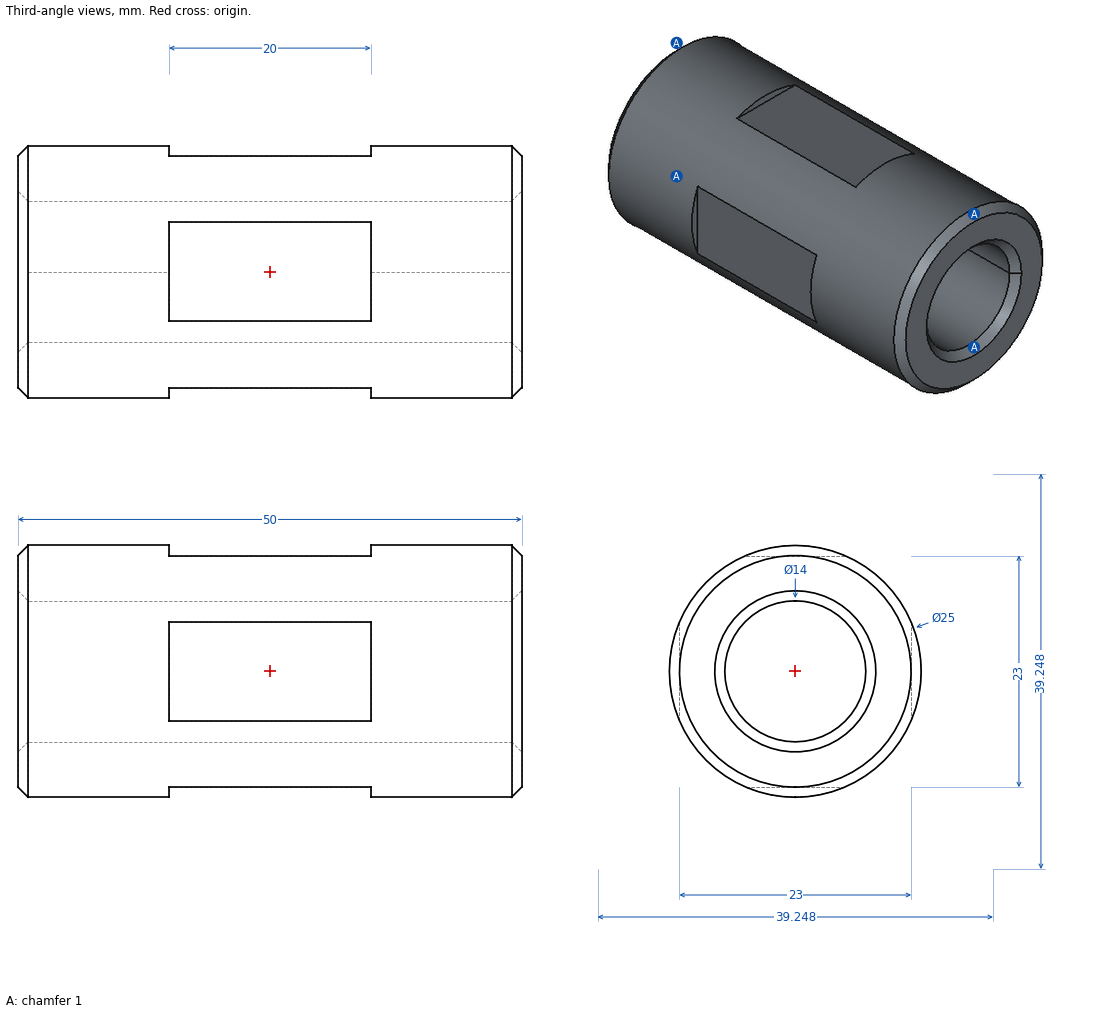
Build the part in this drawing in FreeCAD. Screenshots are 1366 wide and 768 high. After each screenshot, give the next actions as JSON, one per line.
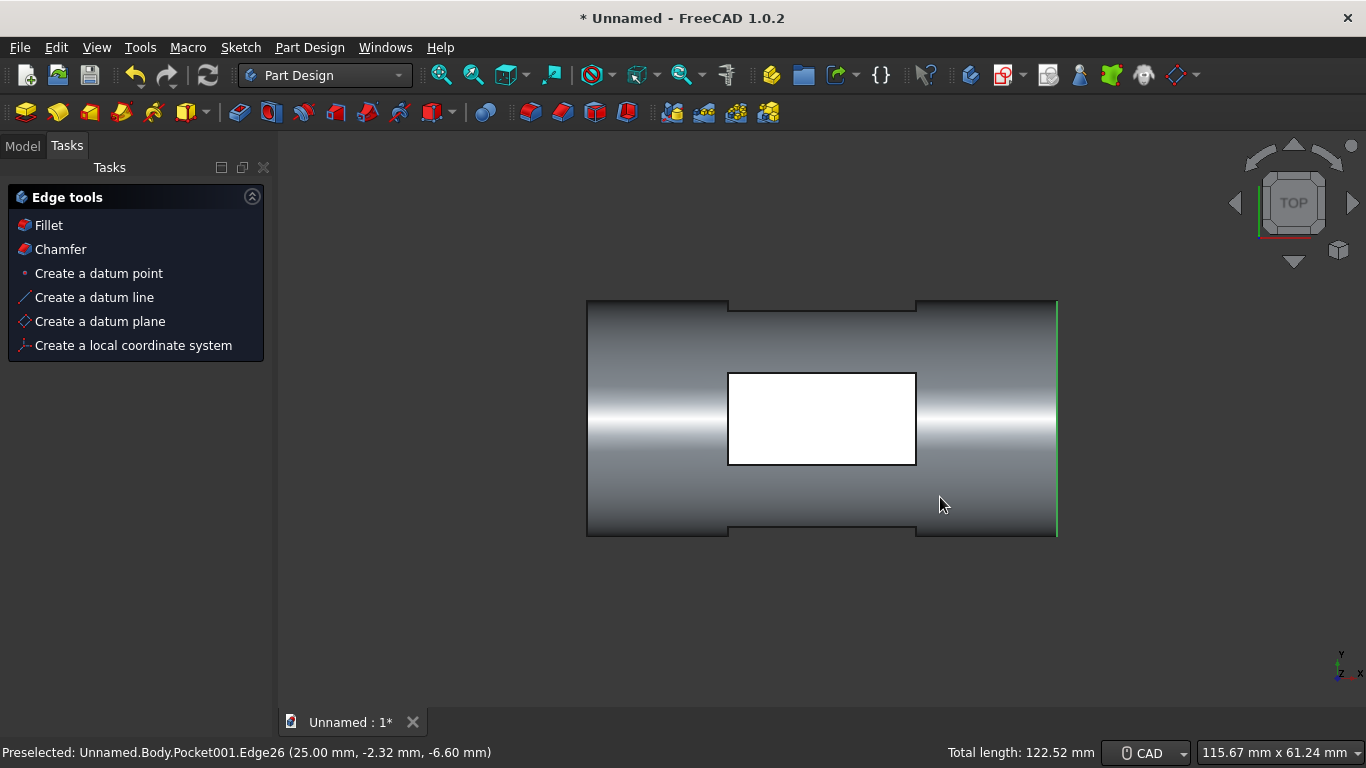
{"action": "left_click", "coordinate": [587, 513], "text": "ctrl"}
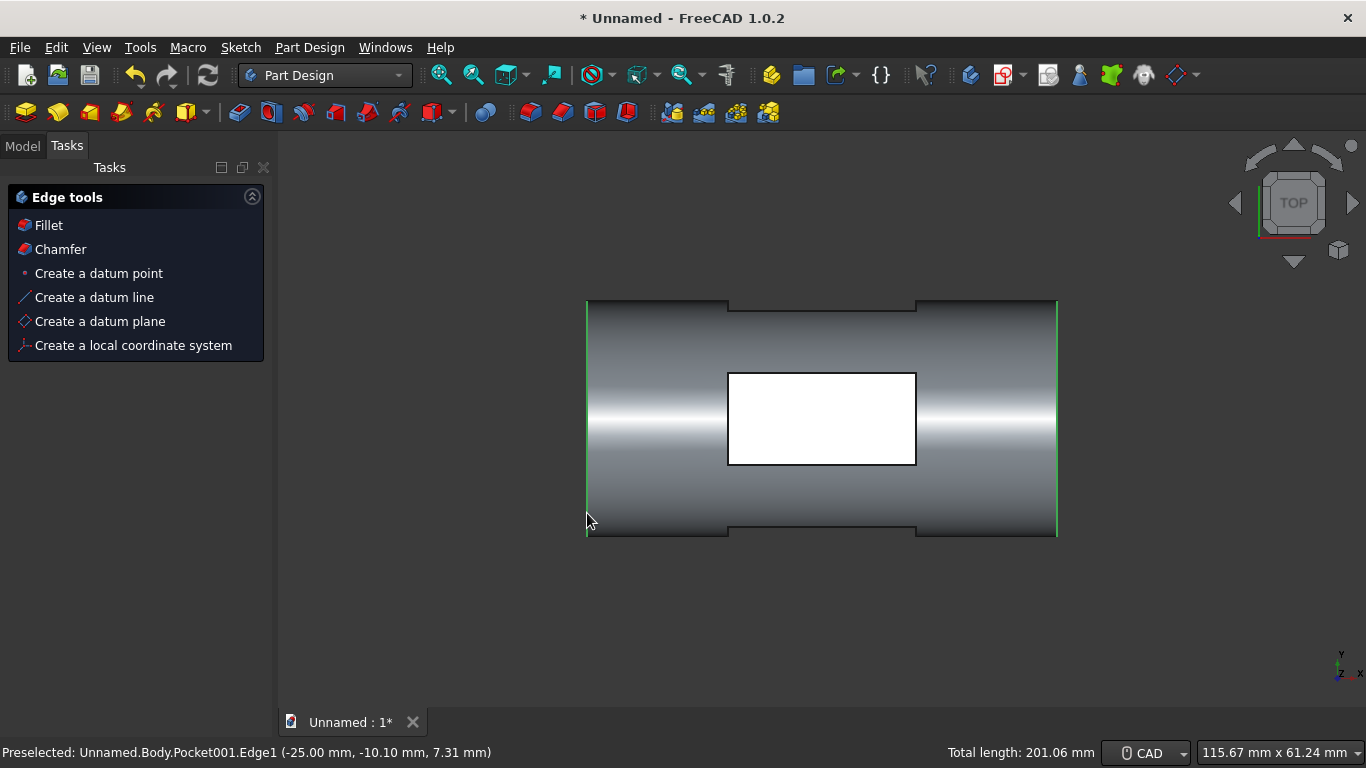
{"action": "key", "text": "1"}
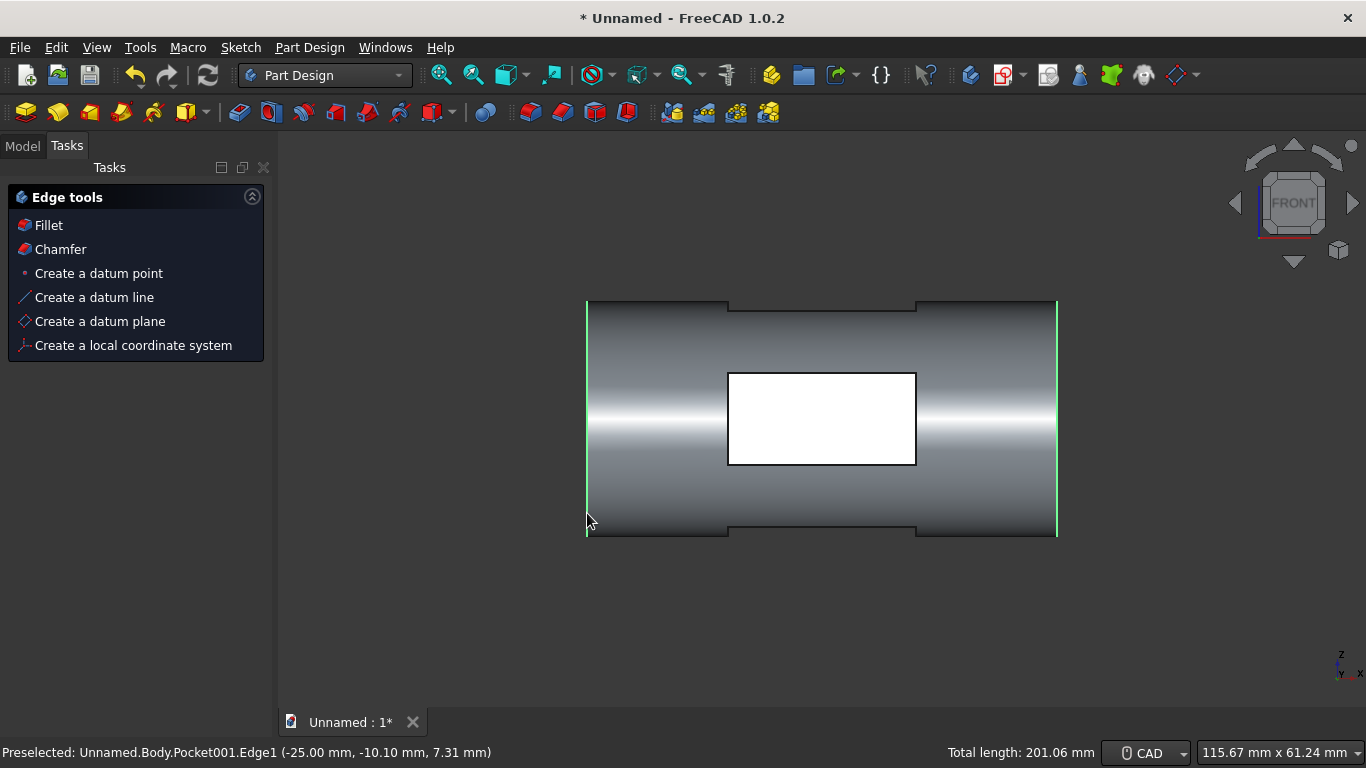
{"action": "left_click", "coordinate": [442, 76]}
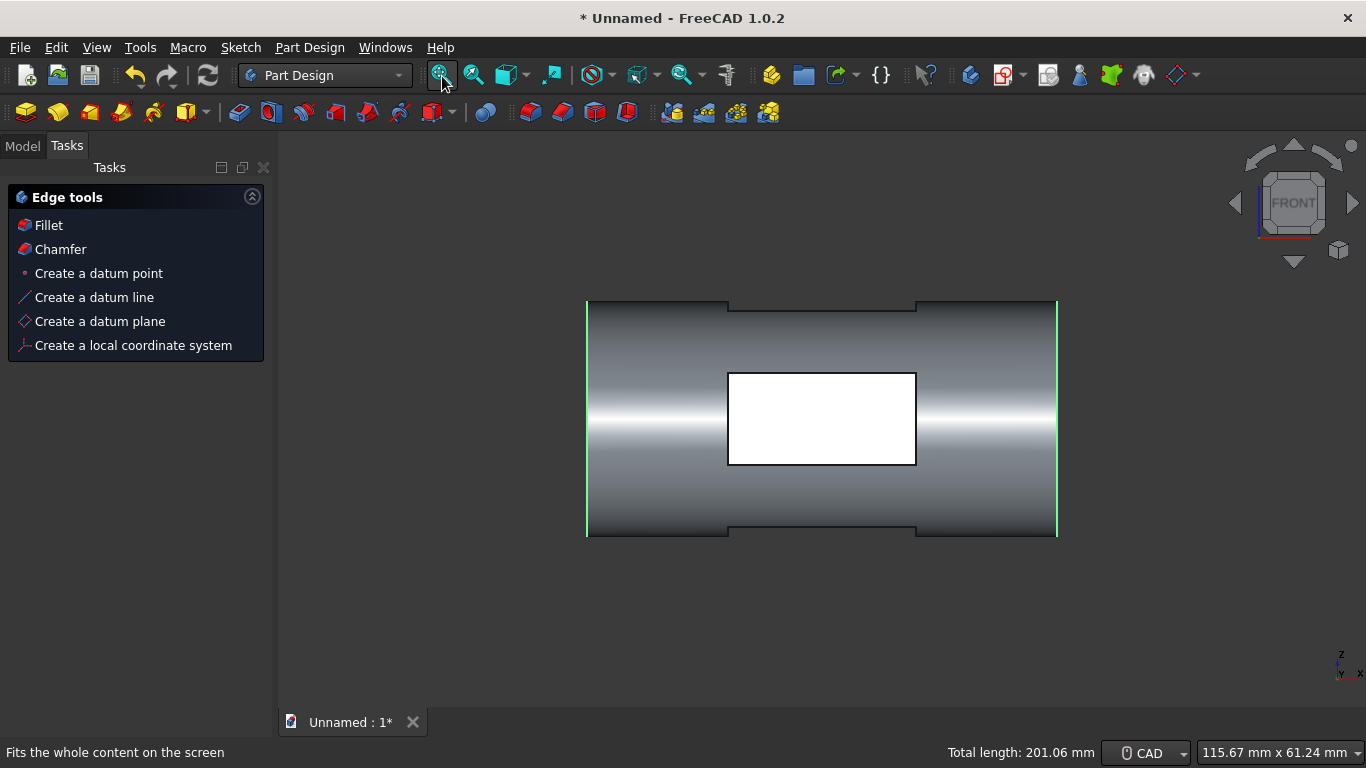
{"action": "key", "text": "3"}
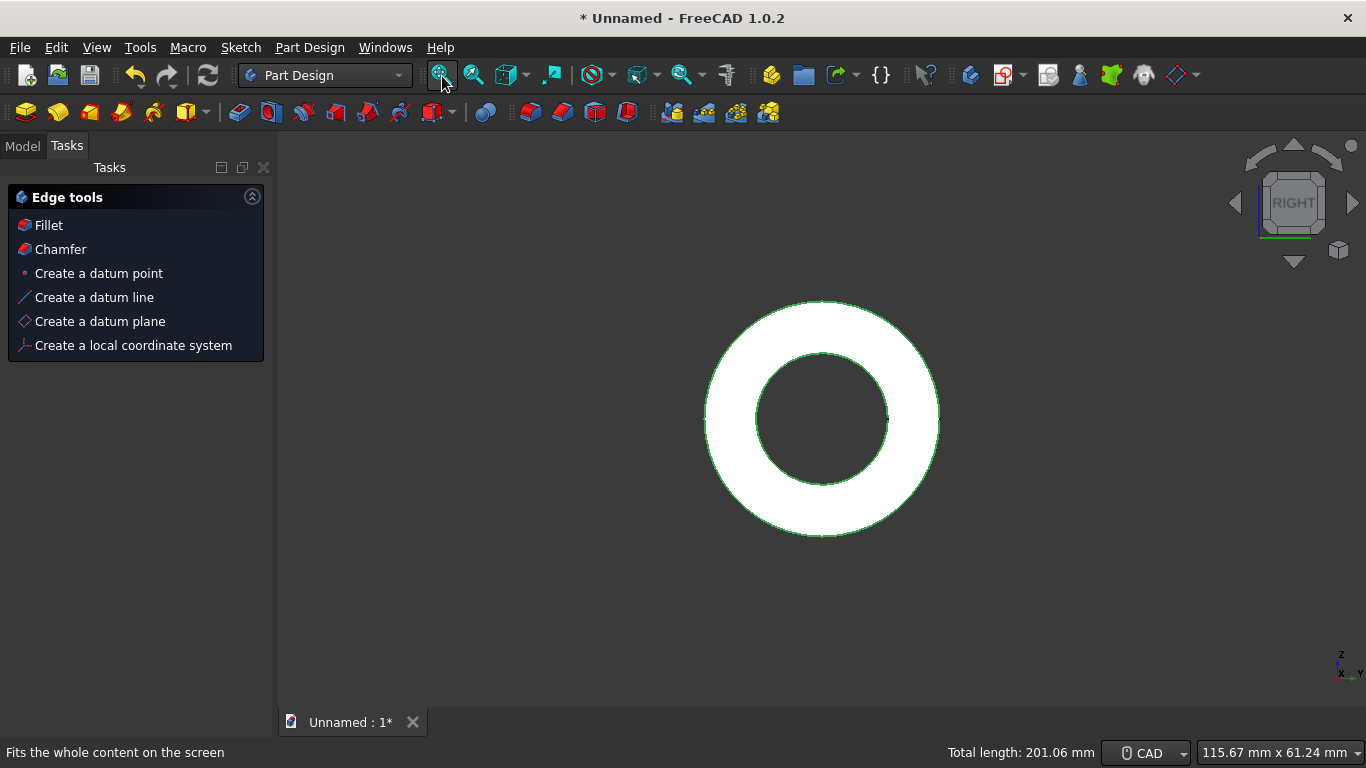
{"action": "left_click", "coordinate": [442, 76]}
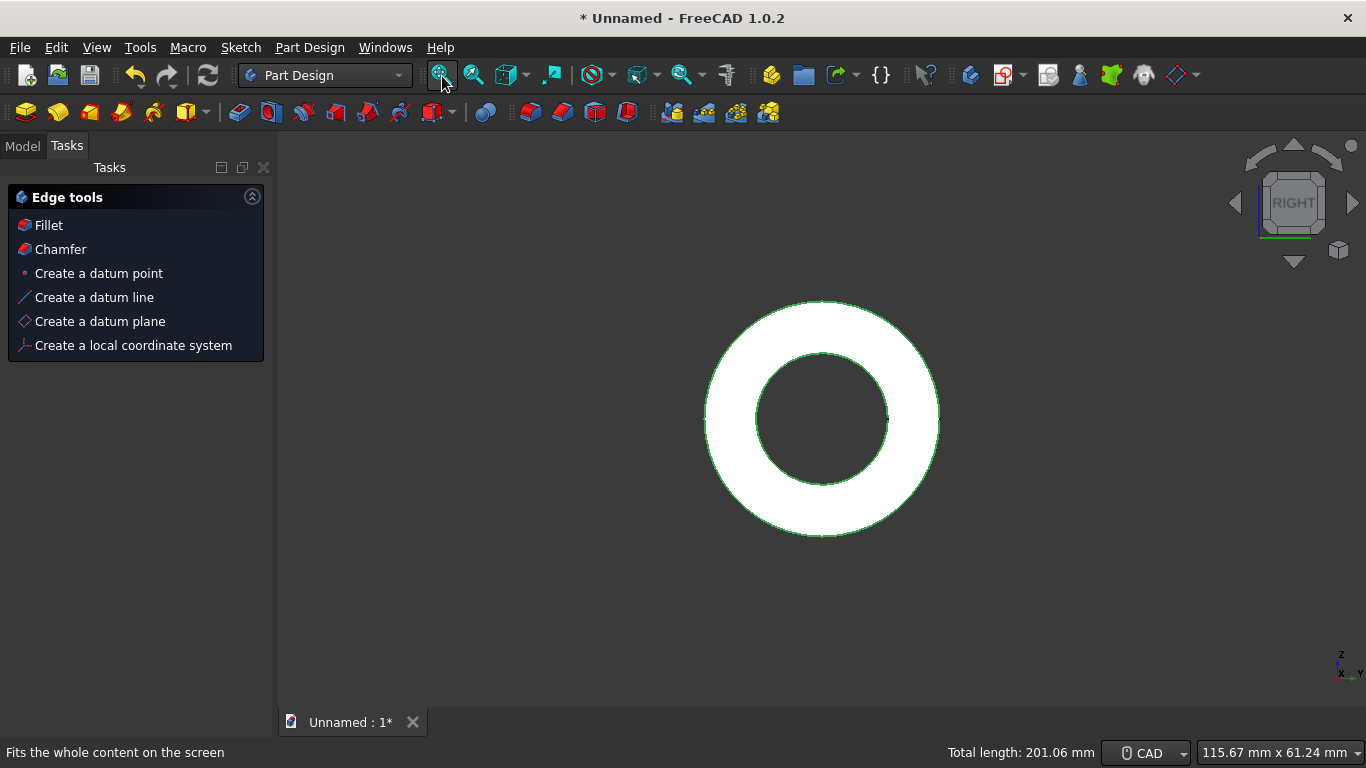
{"action": "key", "text": "5"}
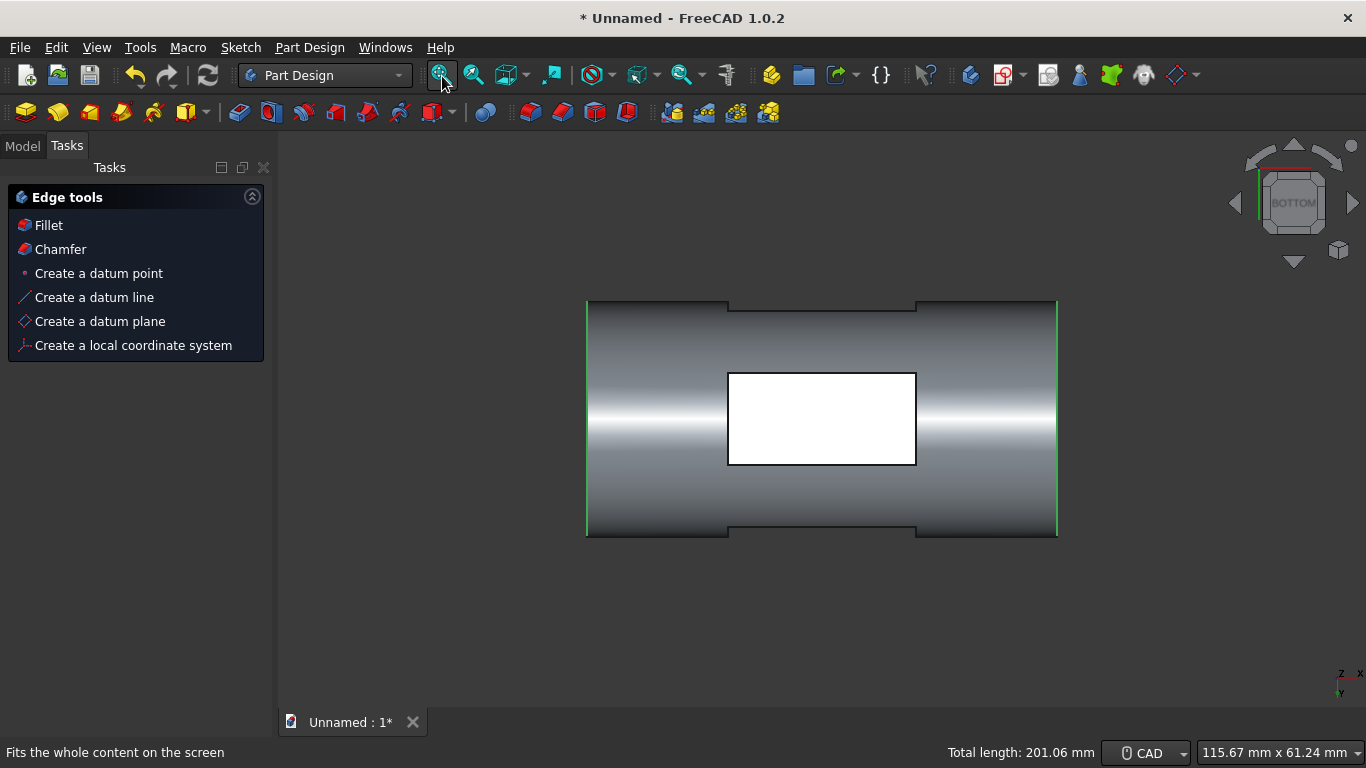
{"action": "left_click", "coordinate": [442, 76]}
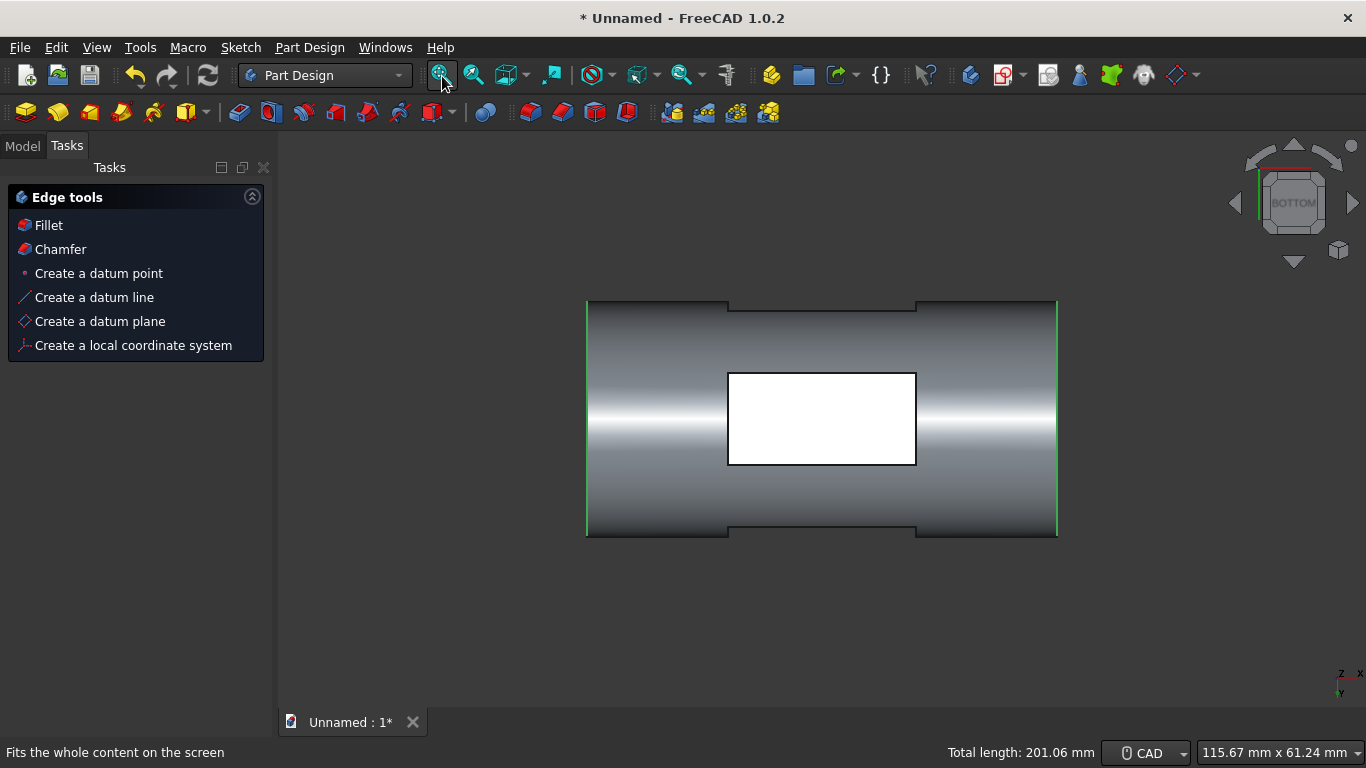
{"action": "key", "text": "4"}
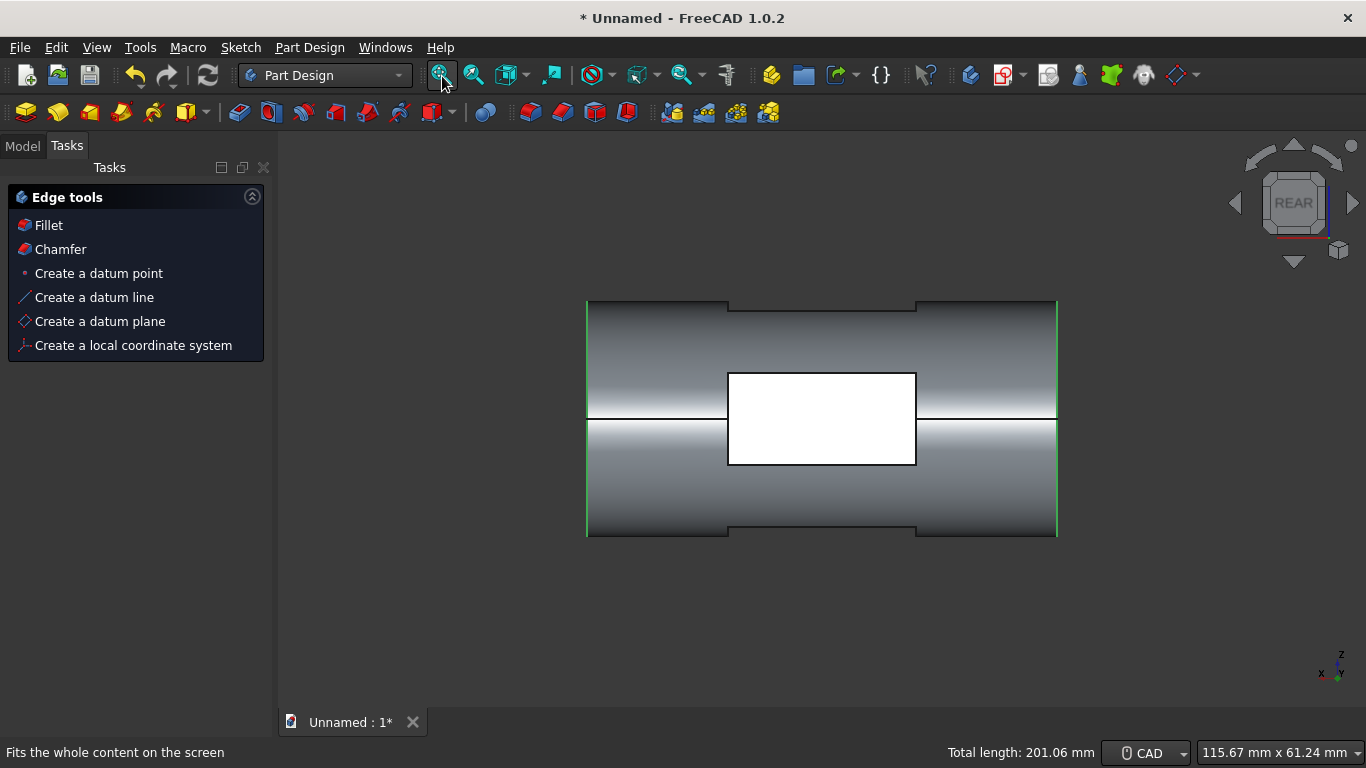
{"action": "left_click", "coordinate": [442, 76]}